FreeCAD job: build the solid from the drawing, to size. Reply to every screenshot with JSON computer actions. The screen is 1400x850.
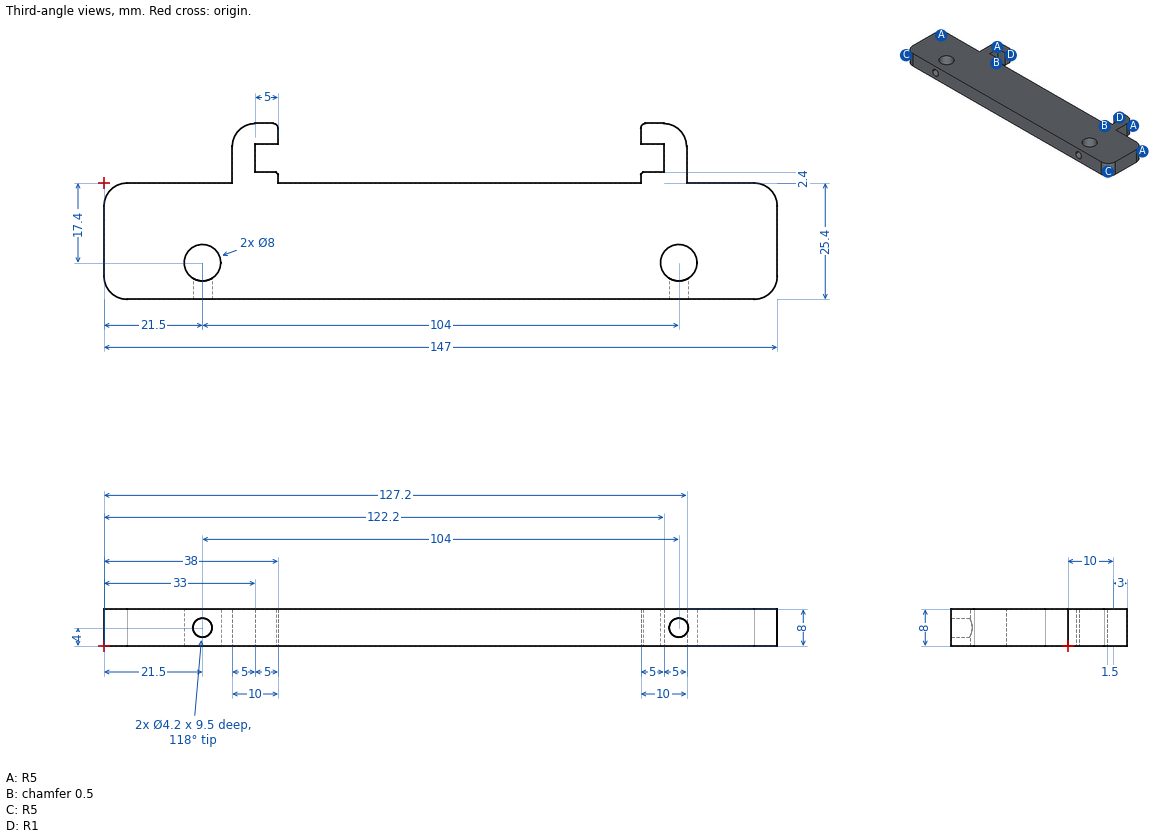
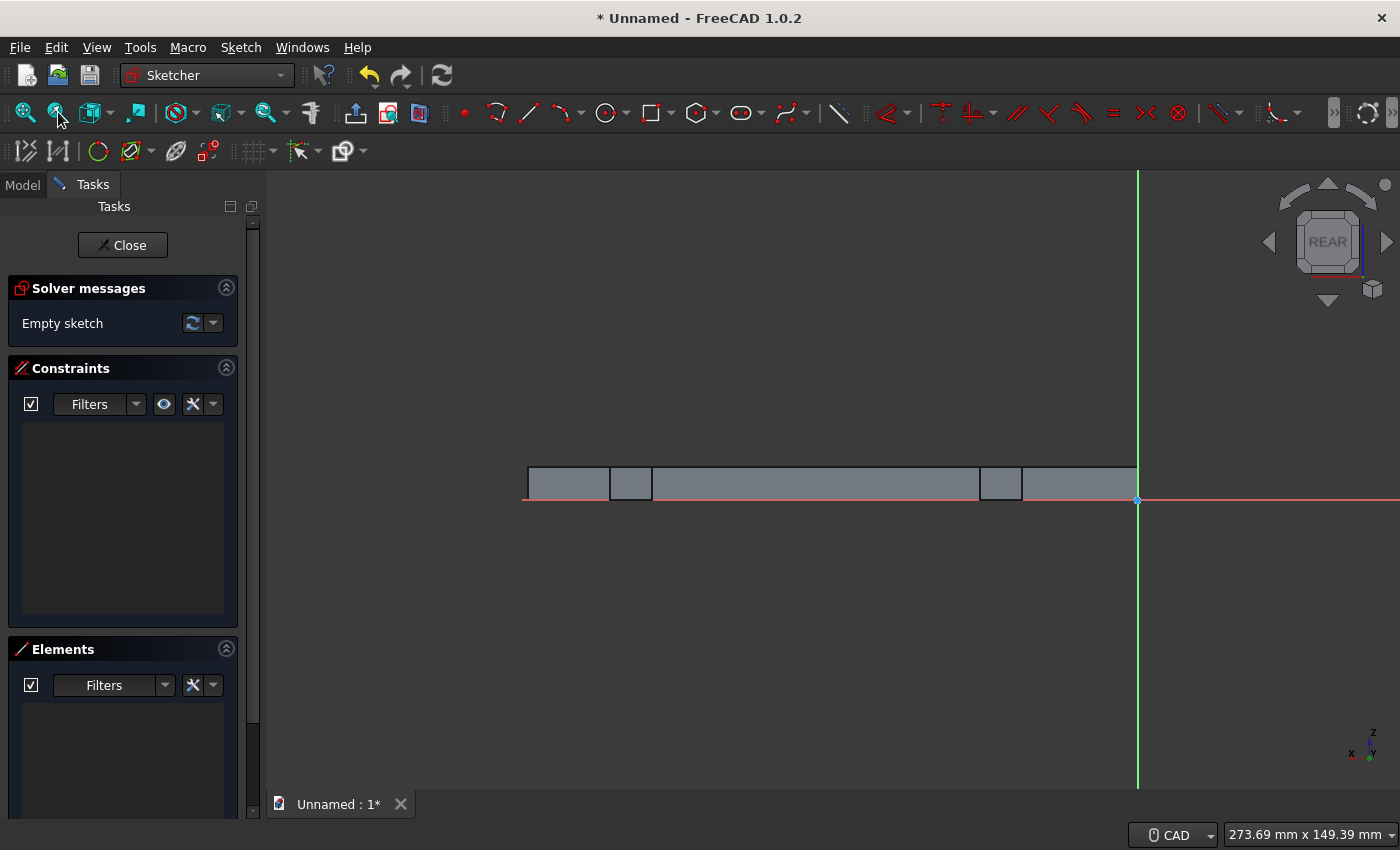
{"action": "left_click", "coordinate": [652, 114]}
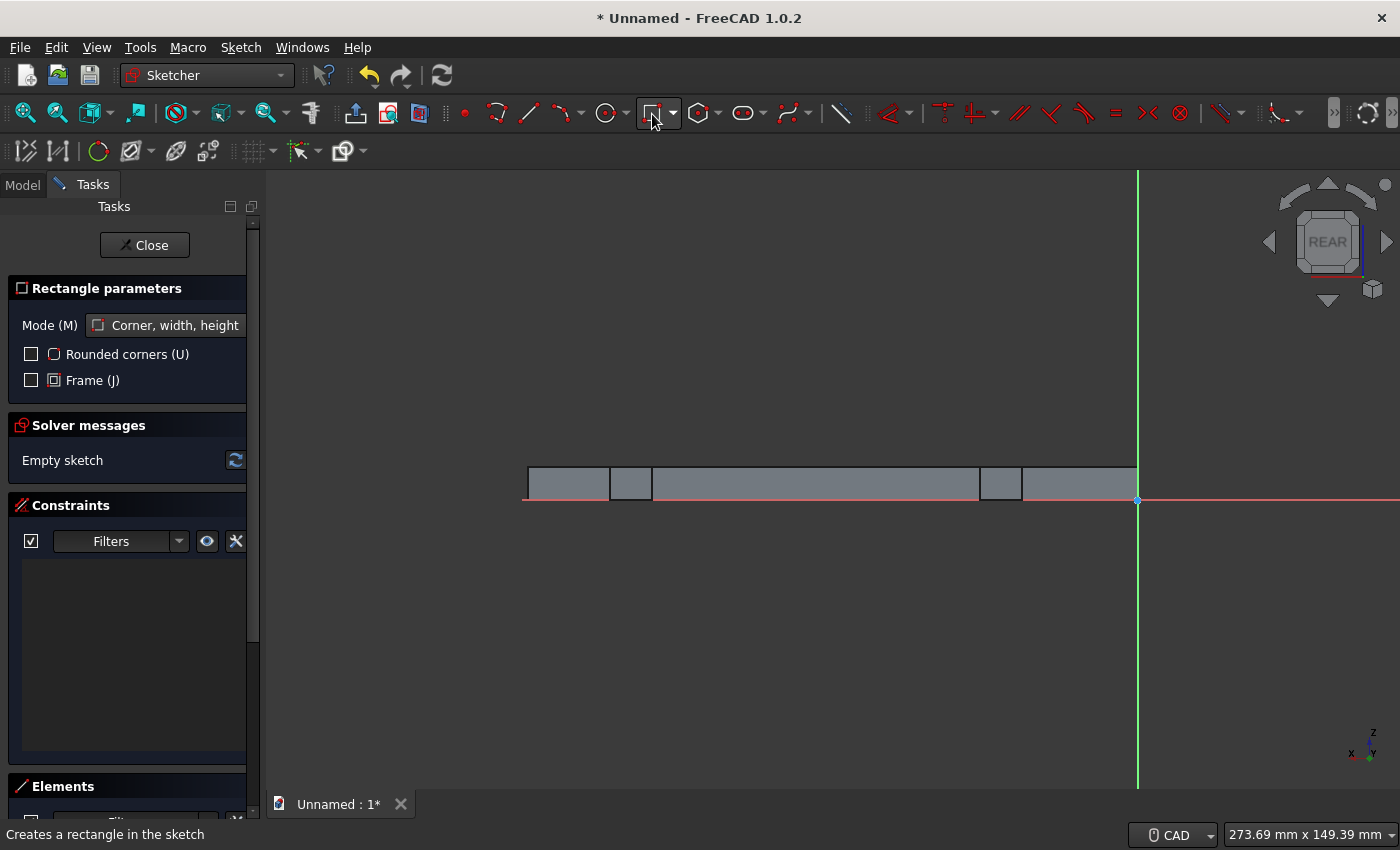
{"action": "left_click", "coordinate": [980, 467]}
{"action": "left_click", "coordinate": [1001, 500]}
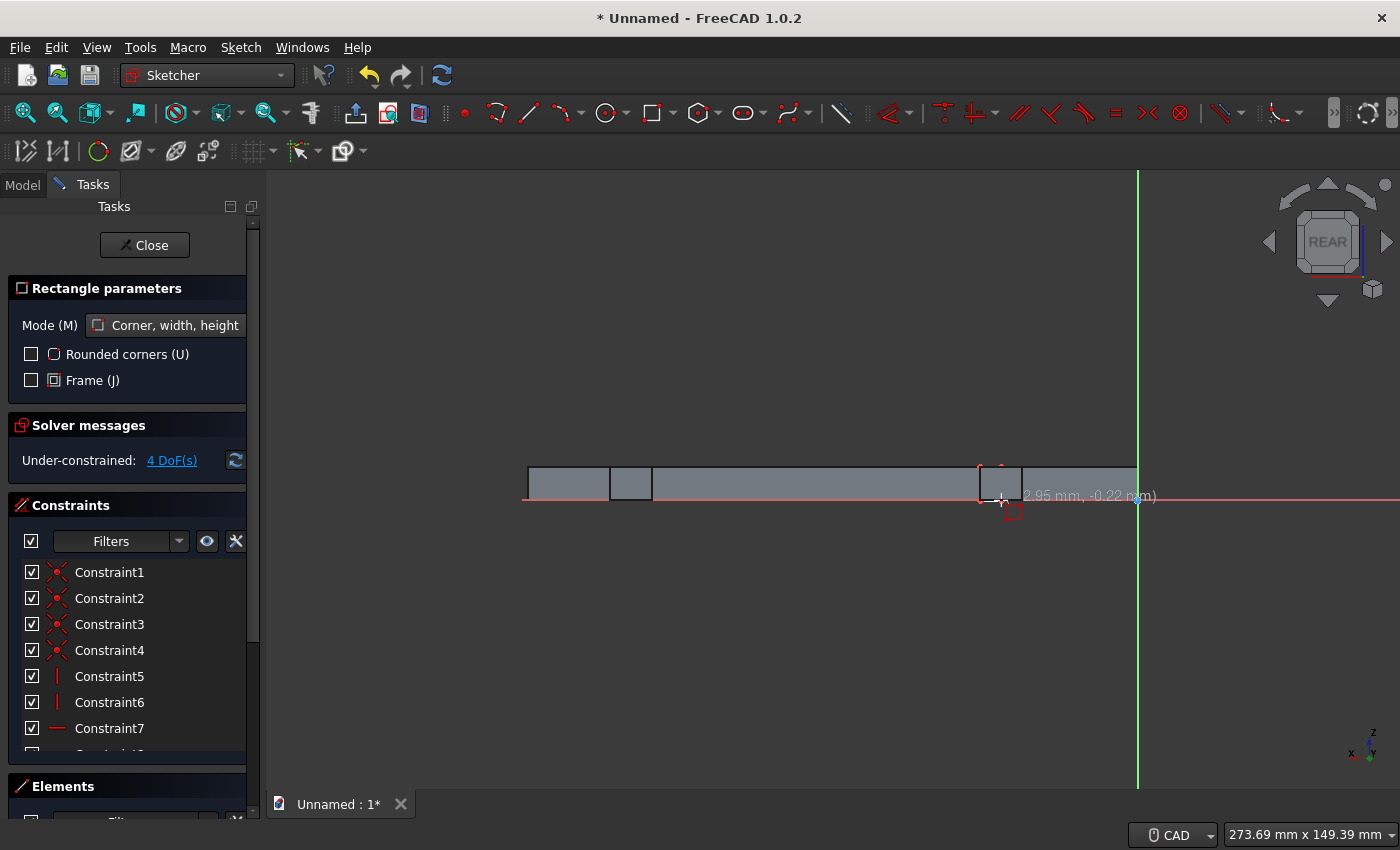
{"action": "left_click", "coordinate": [631, 467]}
{"action": "left_click", "coordinate": [652, 500]}
{"action": "key", "text": "Escape"}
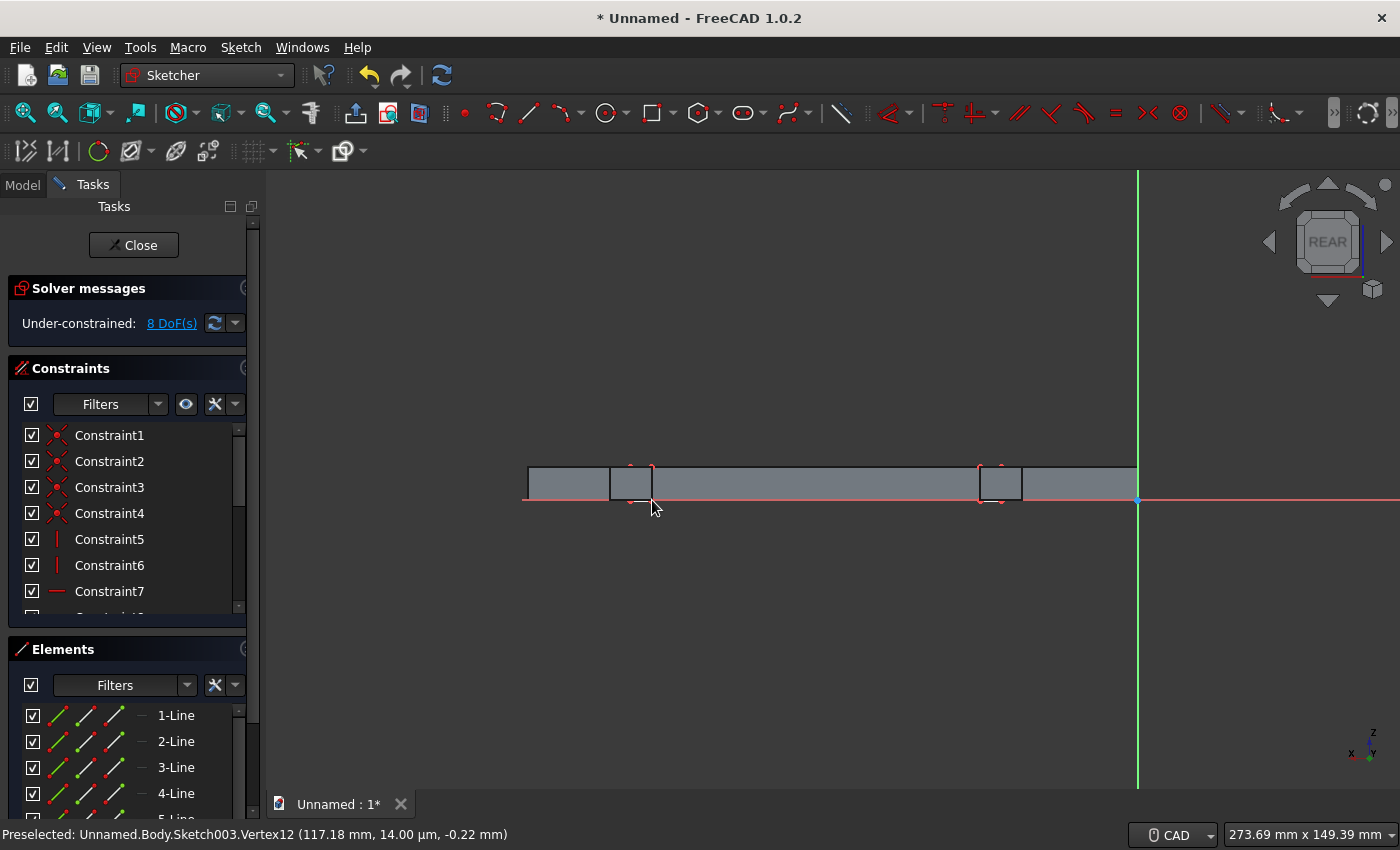
{"action": "left_click", "coordinate": [980, 501]}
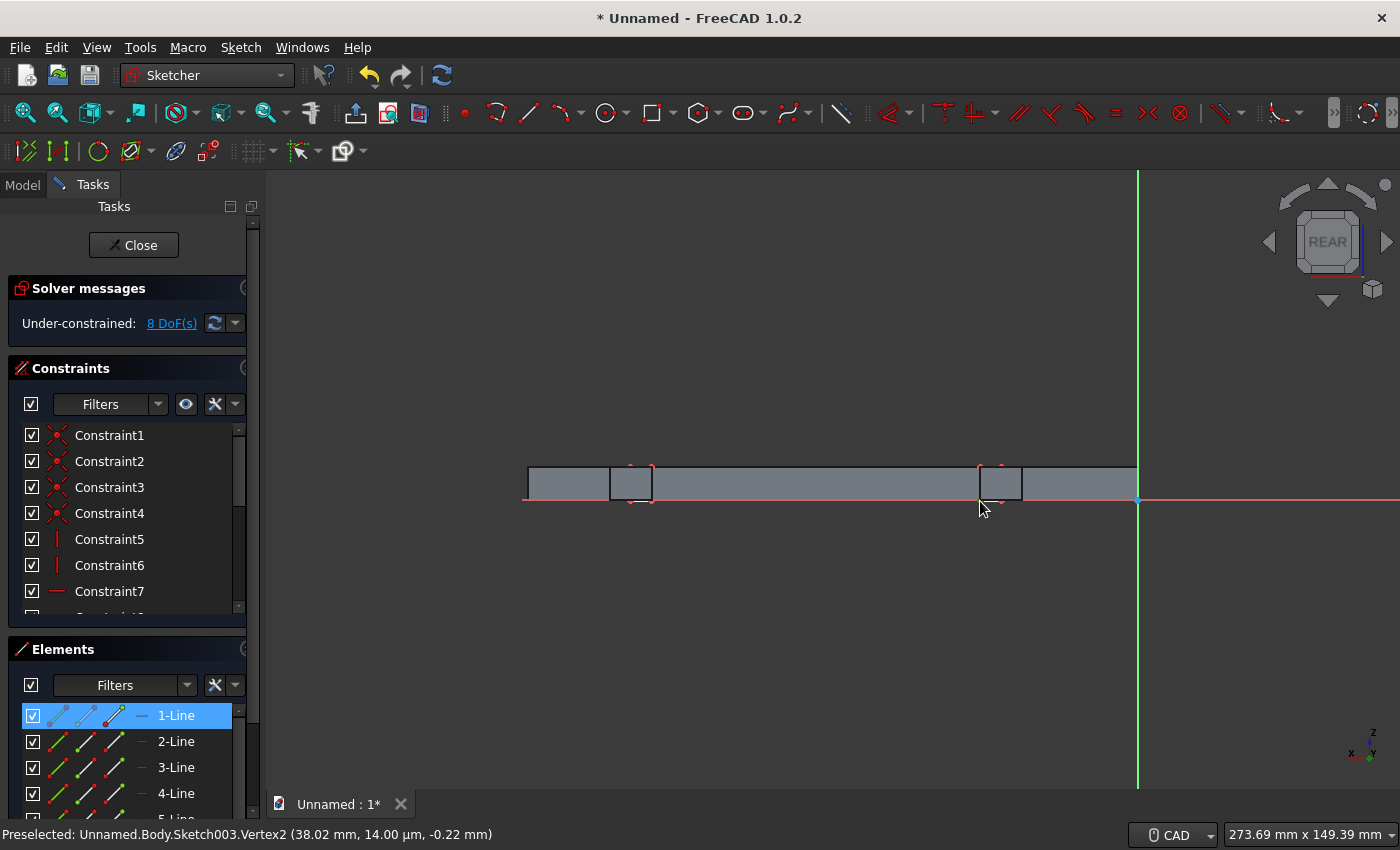
{"action": "left_click", "coordinate": [563, 500]}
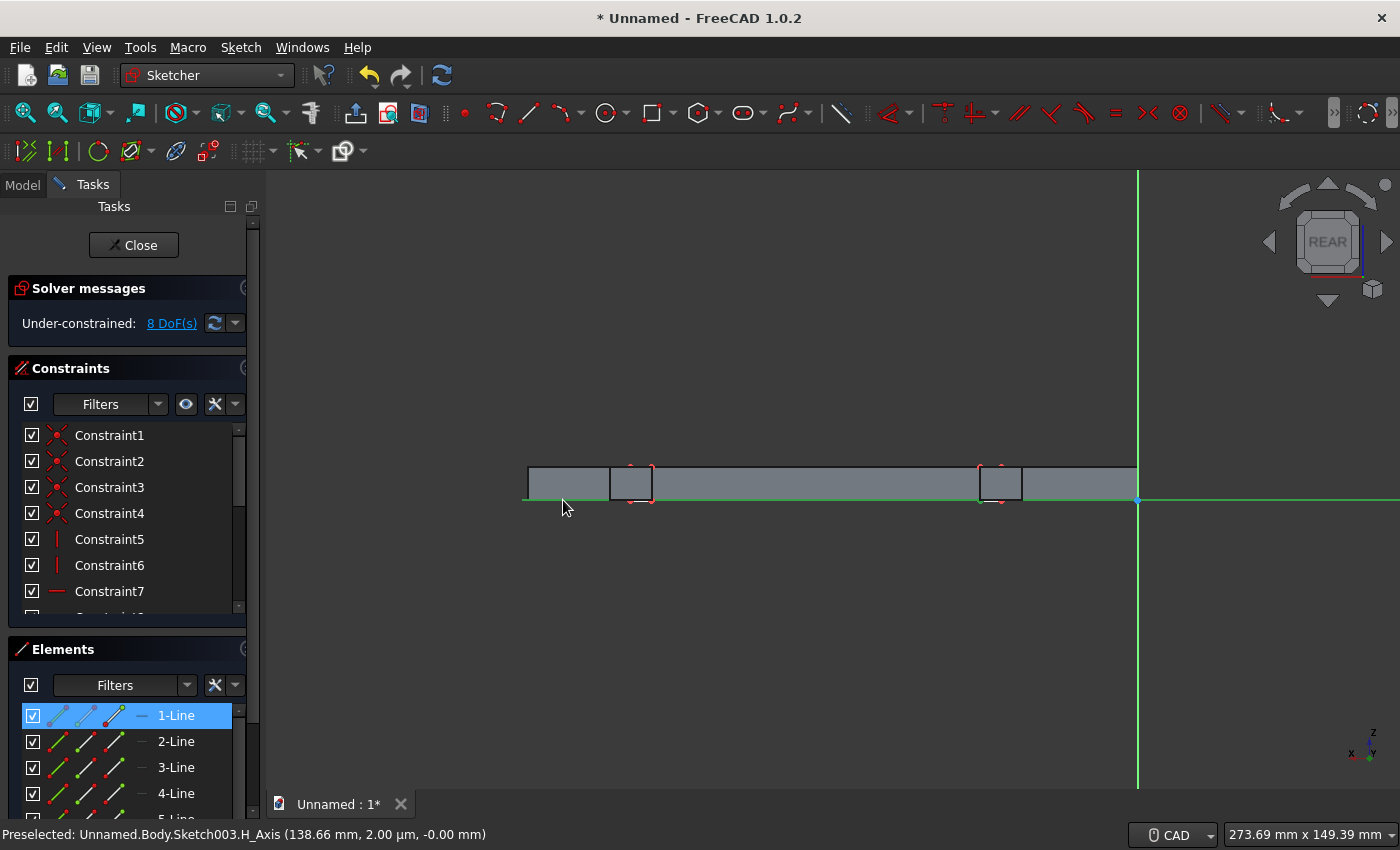
{"action": "left_click", "coordinate": [944, 114]}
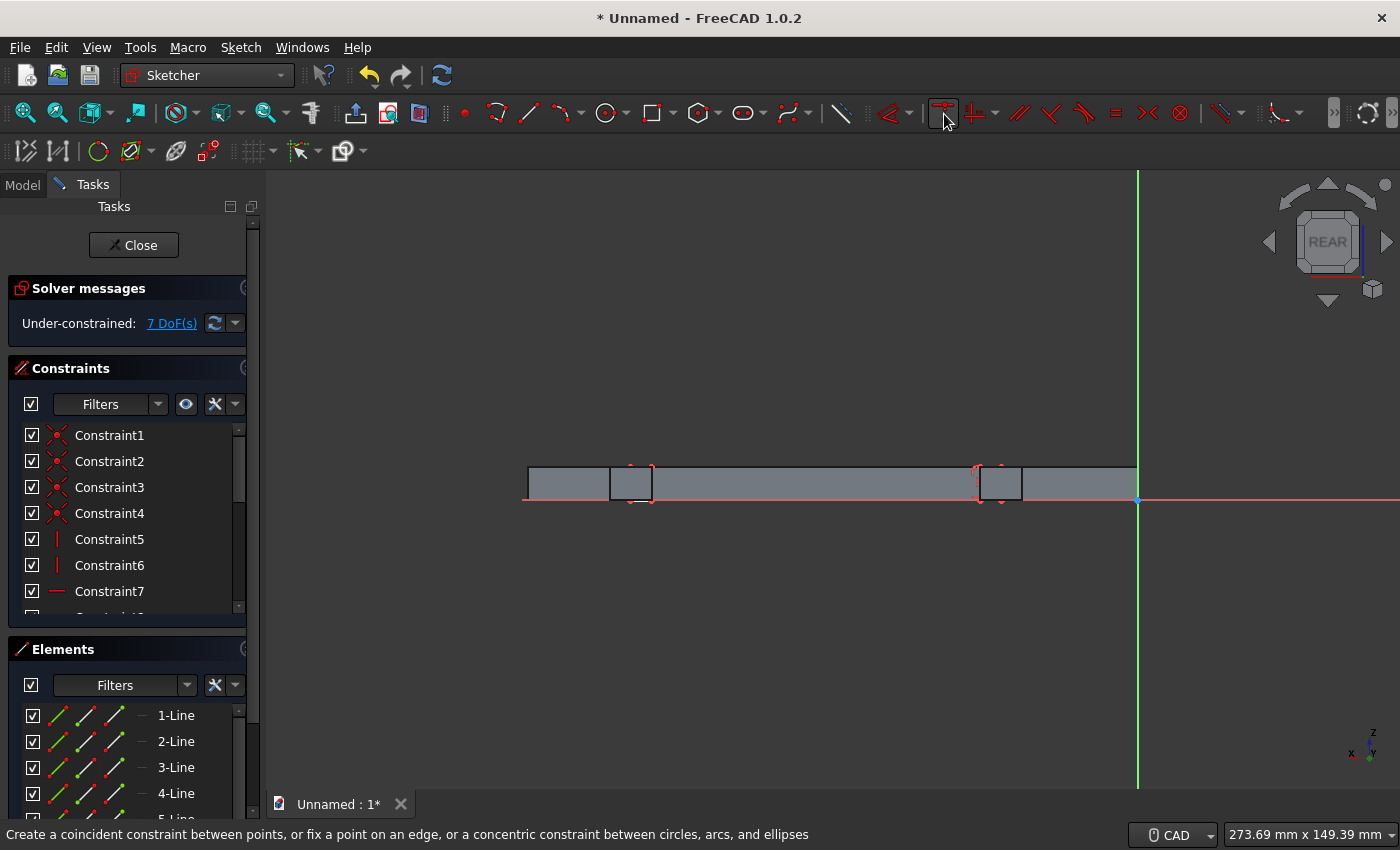
{"action": "left_click", "coordinate": [631, 501]}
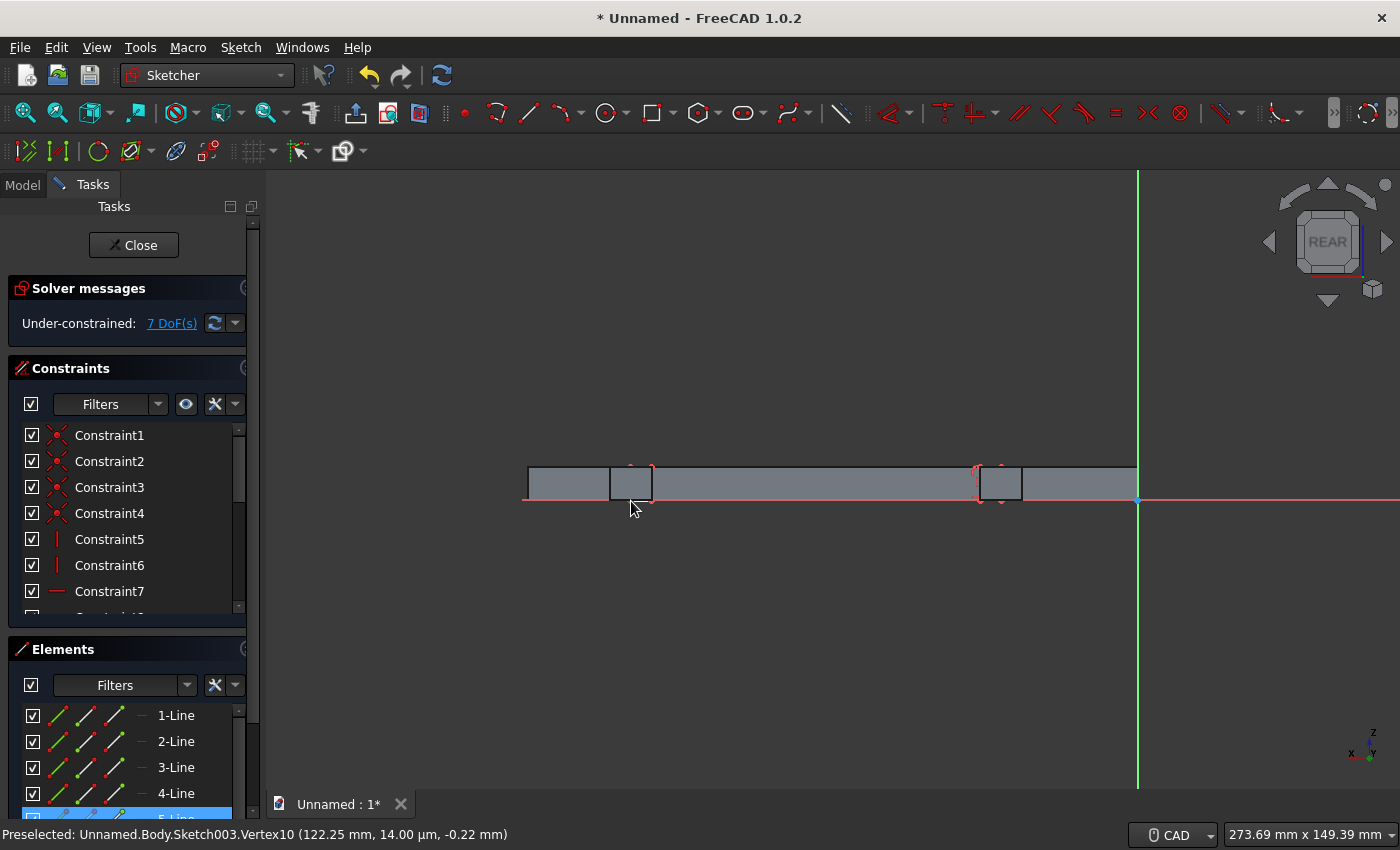
{"action": "left_click", "coordinate": [563, 500]}